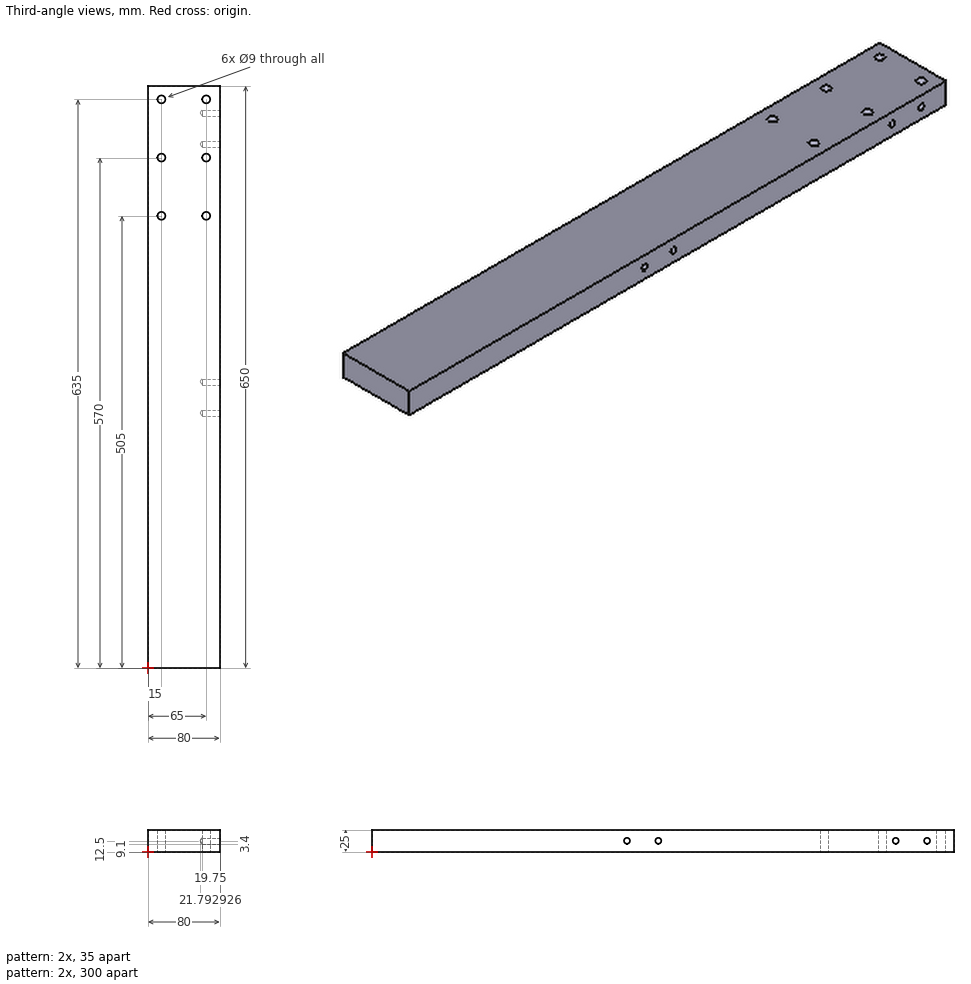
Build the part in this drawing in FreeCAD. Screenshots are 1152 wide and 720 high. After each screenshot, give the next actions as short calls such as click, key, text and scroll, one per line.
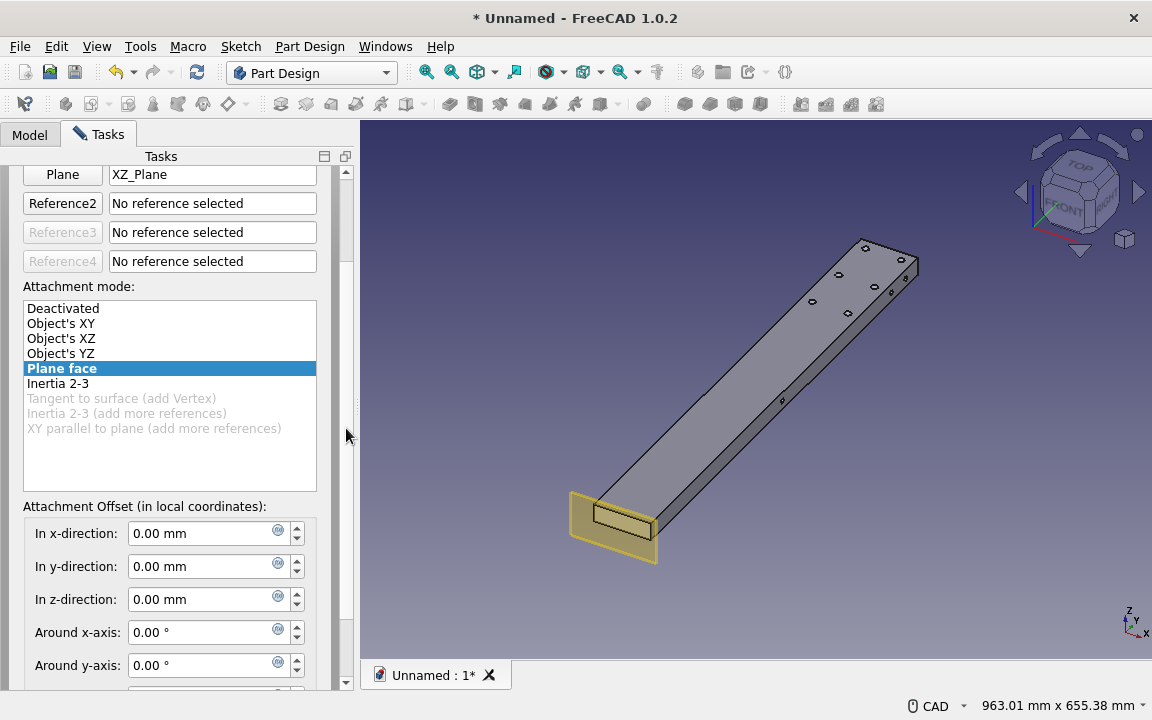
triple_click(210, 600)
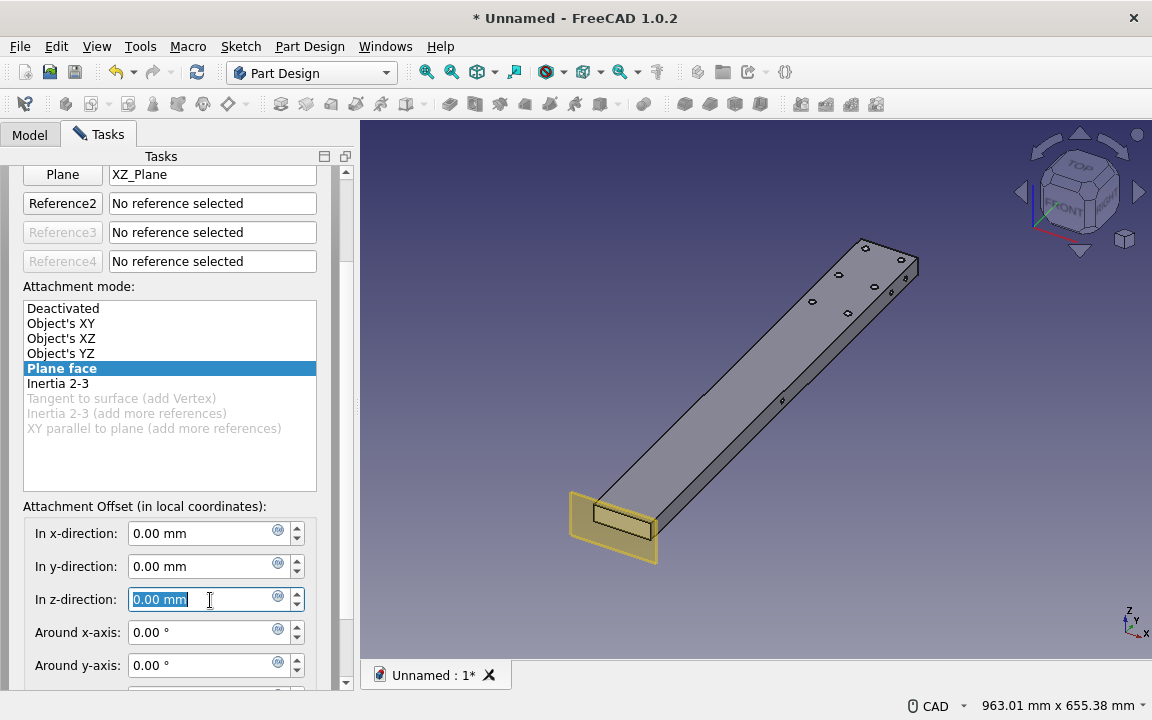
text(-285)
key(Tab)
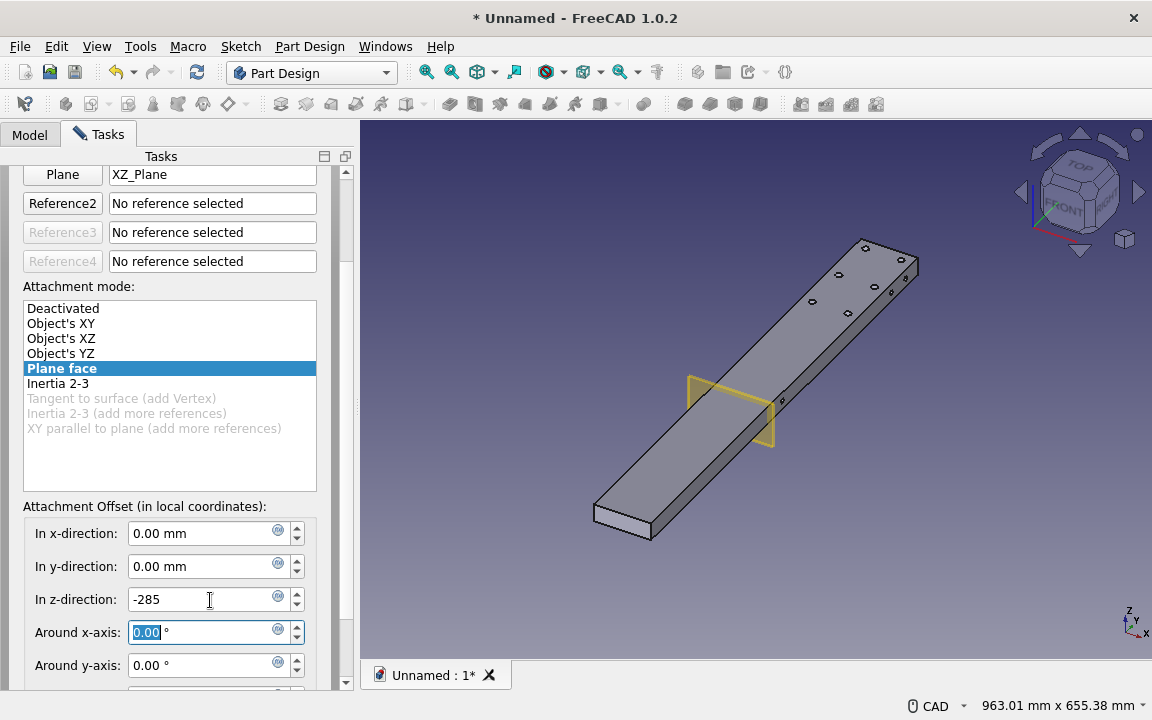
scroll(346, 428, up, 3)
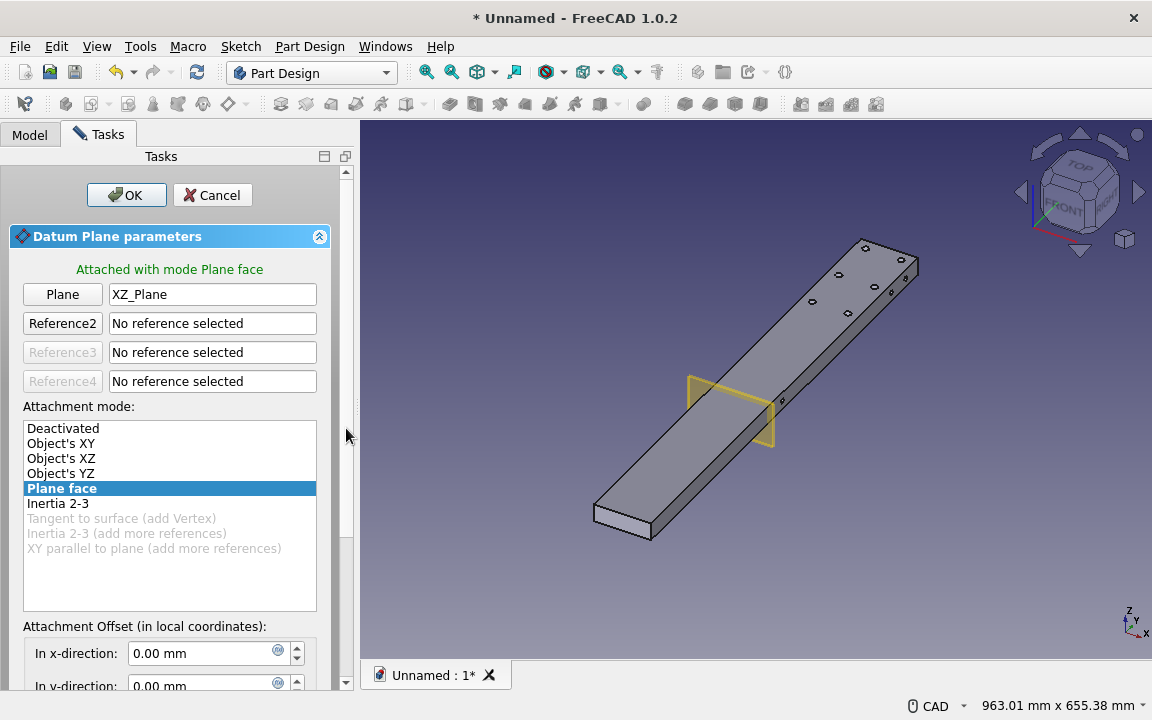
click(127, 195)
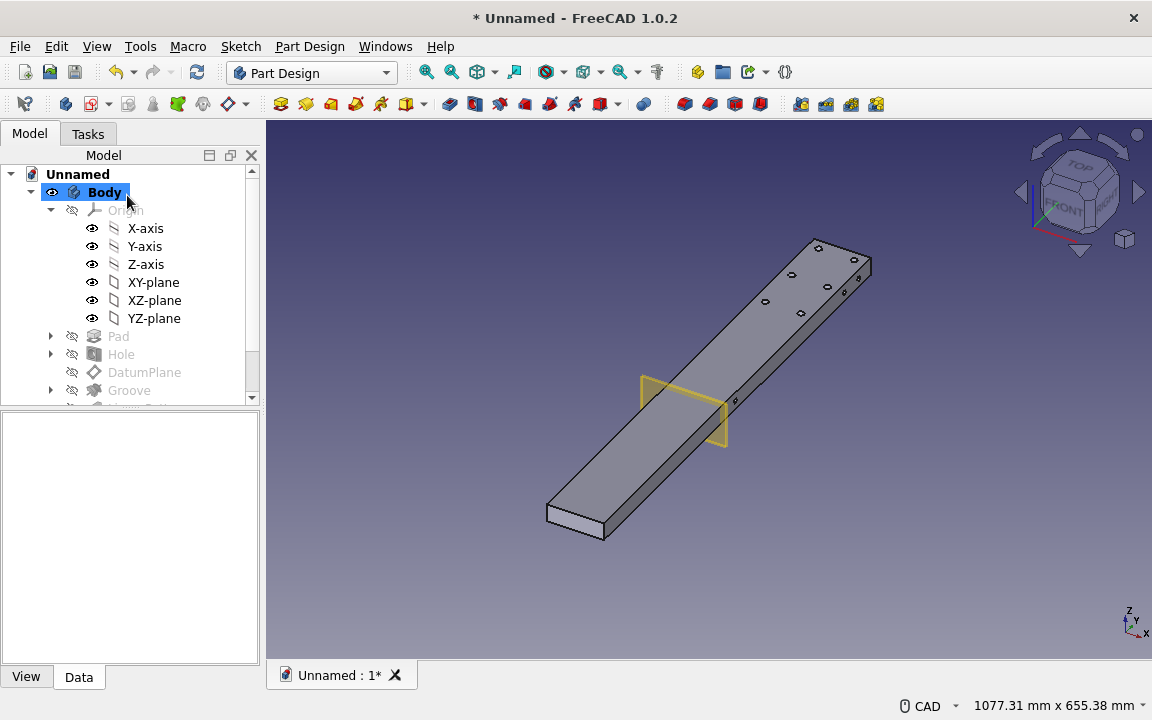
scroll(101, 278, down, 3)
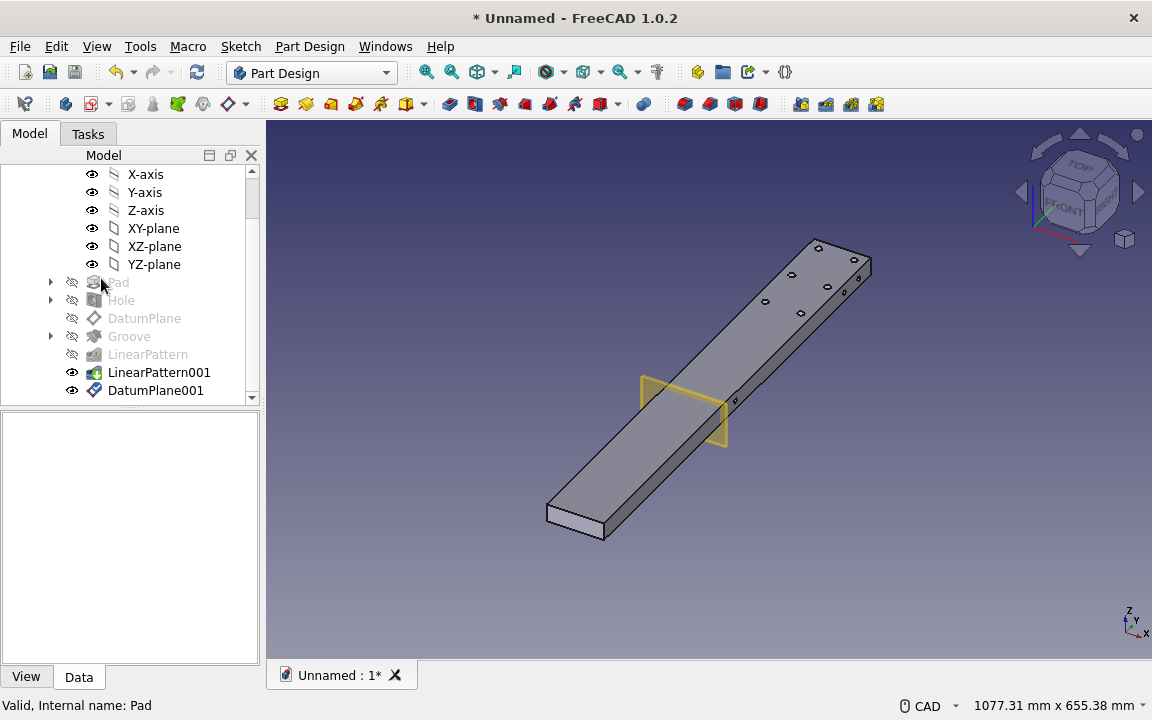
click(117, 390)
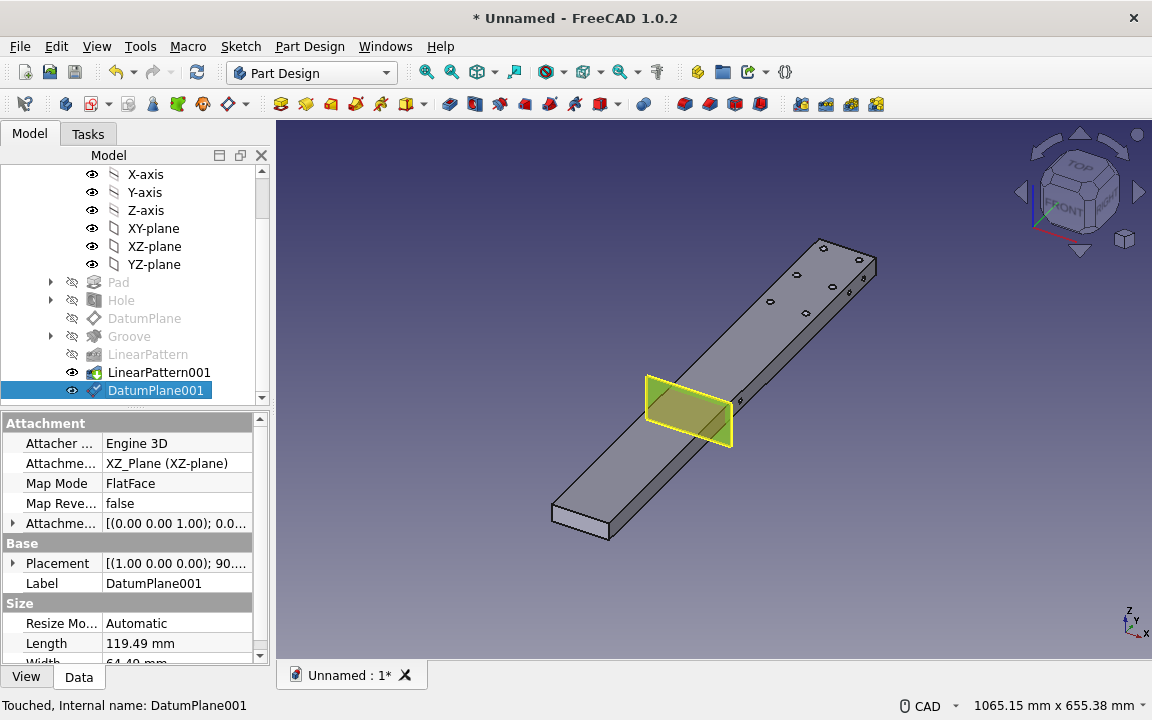
click(90, 104)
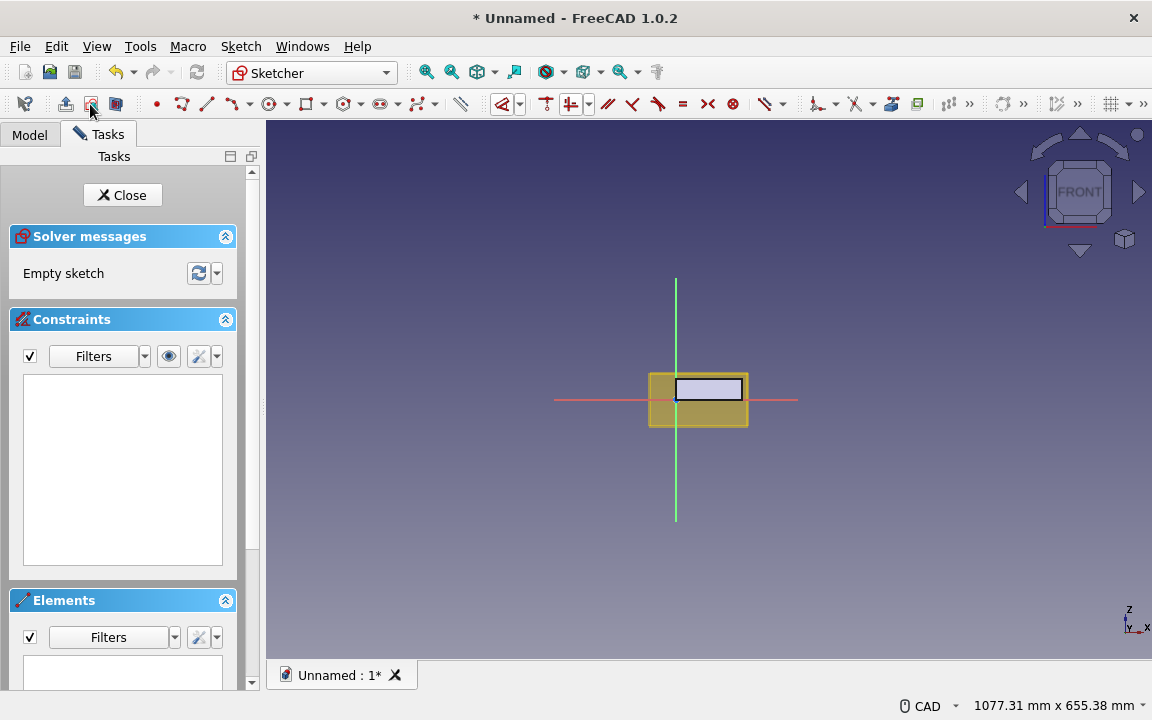
key(q)
key(s)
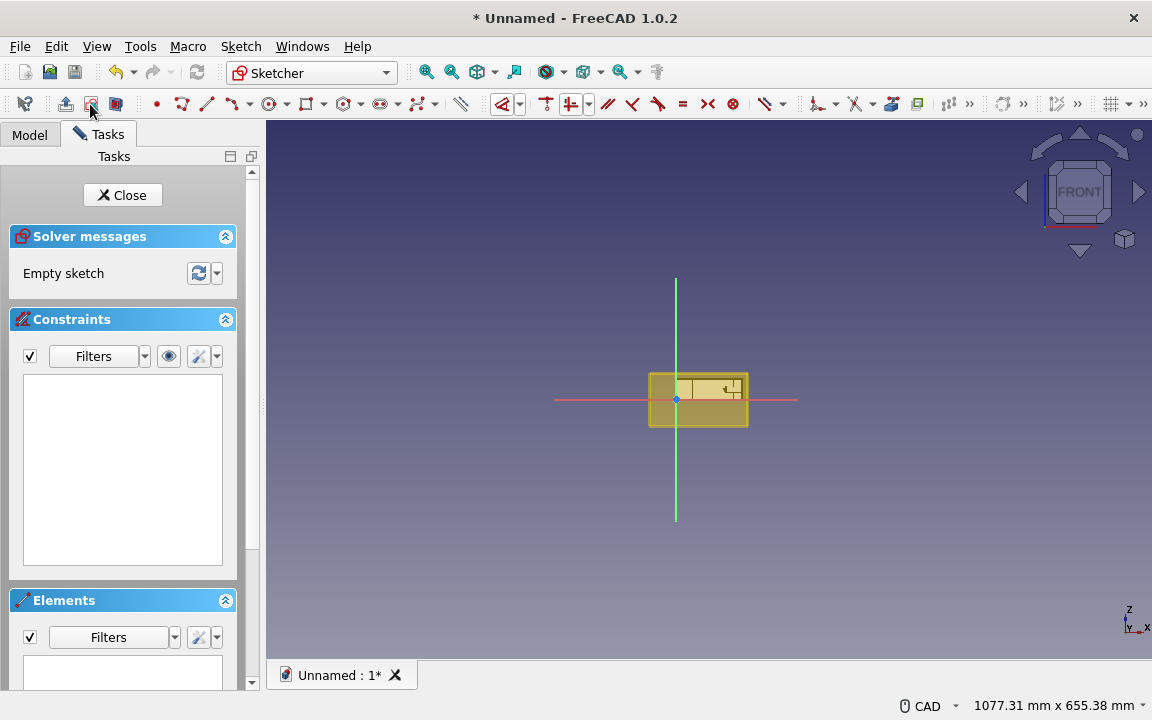
scroll(734, 391, up, 15)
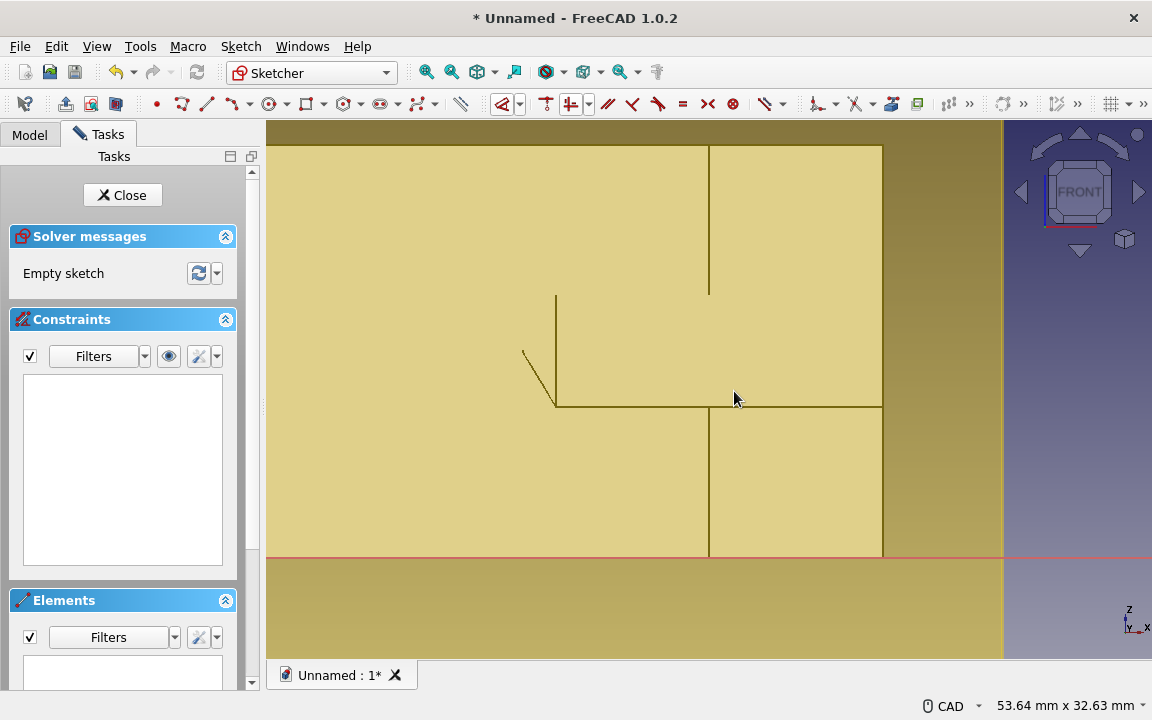
click(182, 104)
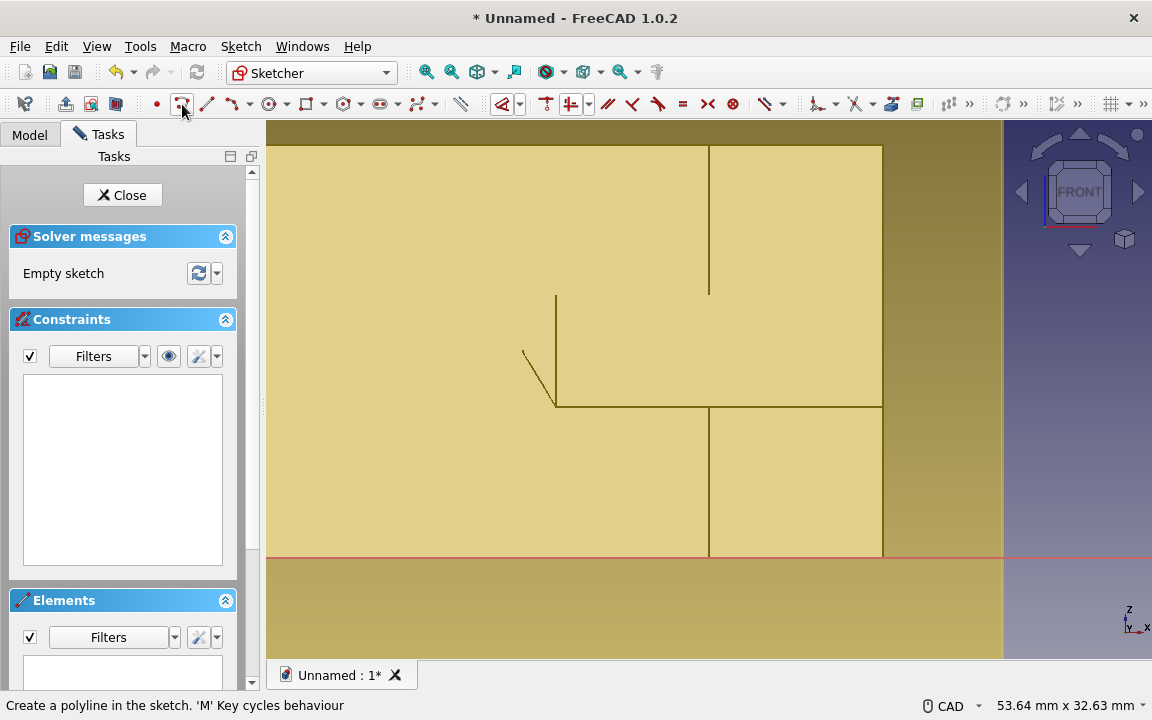
click(523, 351)
click(883, 351)
click(883, 407)
click(556, 407)
click(523, 352)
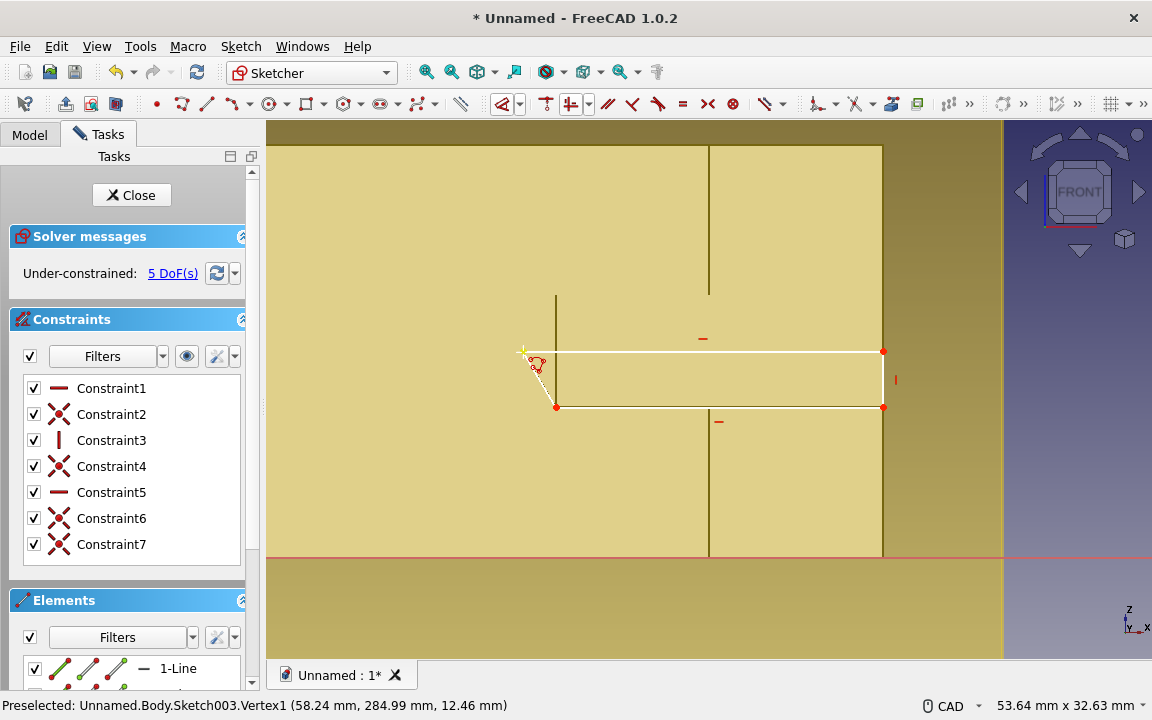
key(g)
key(l)